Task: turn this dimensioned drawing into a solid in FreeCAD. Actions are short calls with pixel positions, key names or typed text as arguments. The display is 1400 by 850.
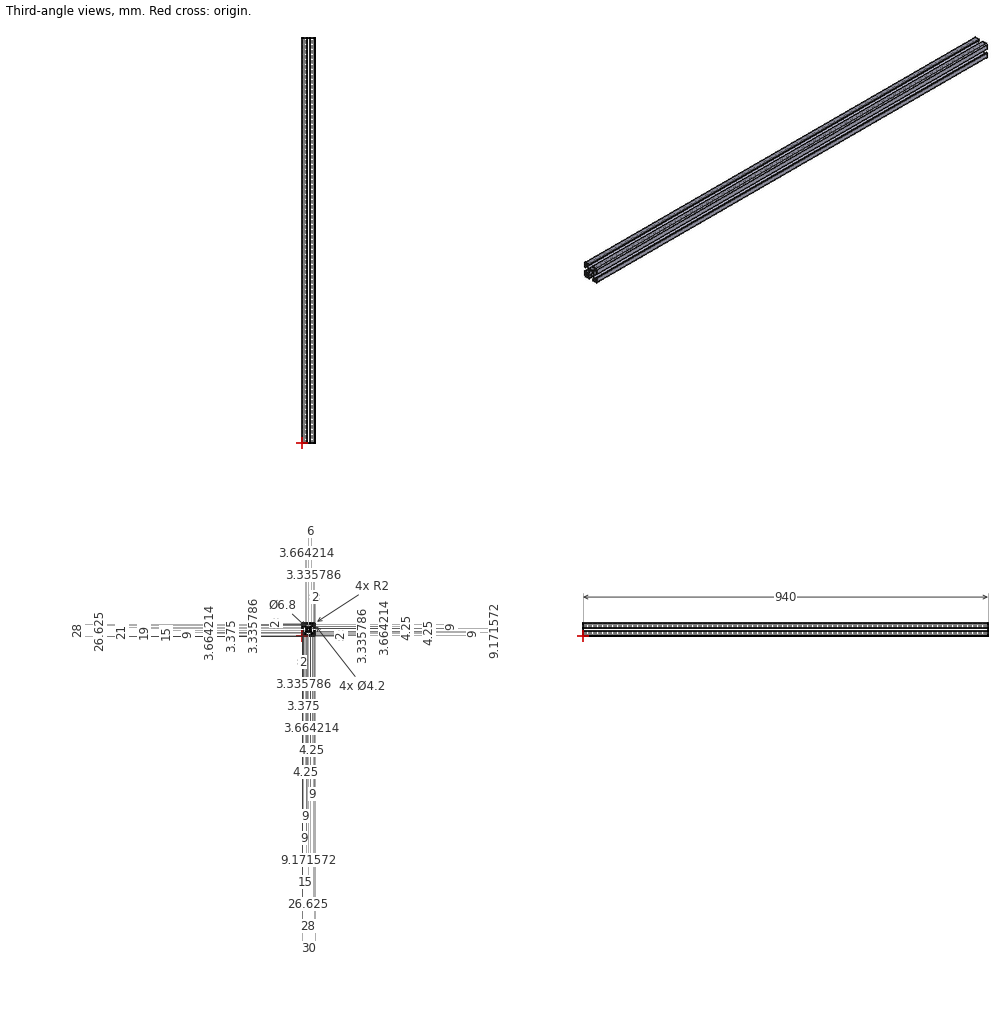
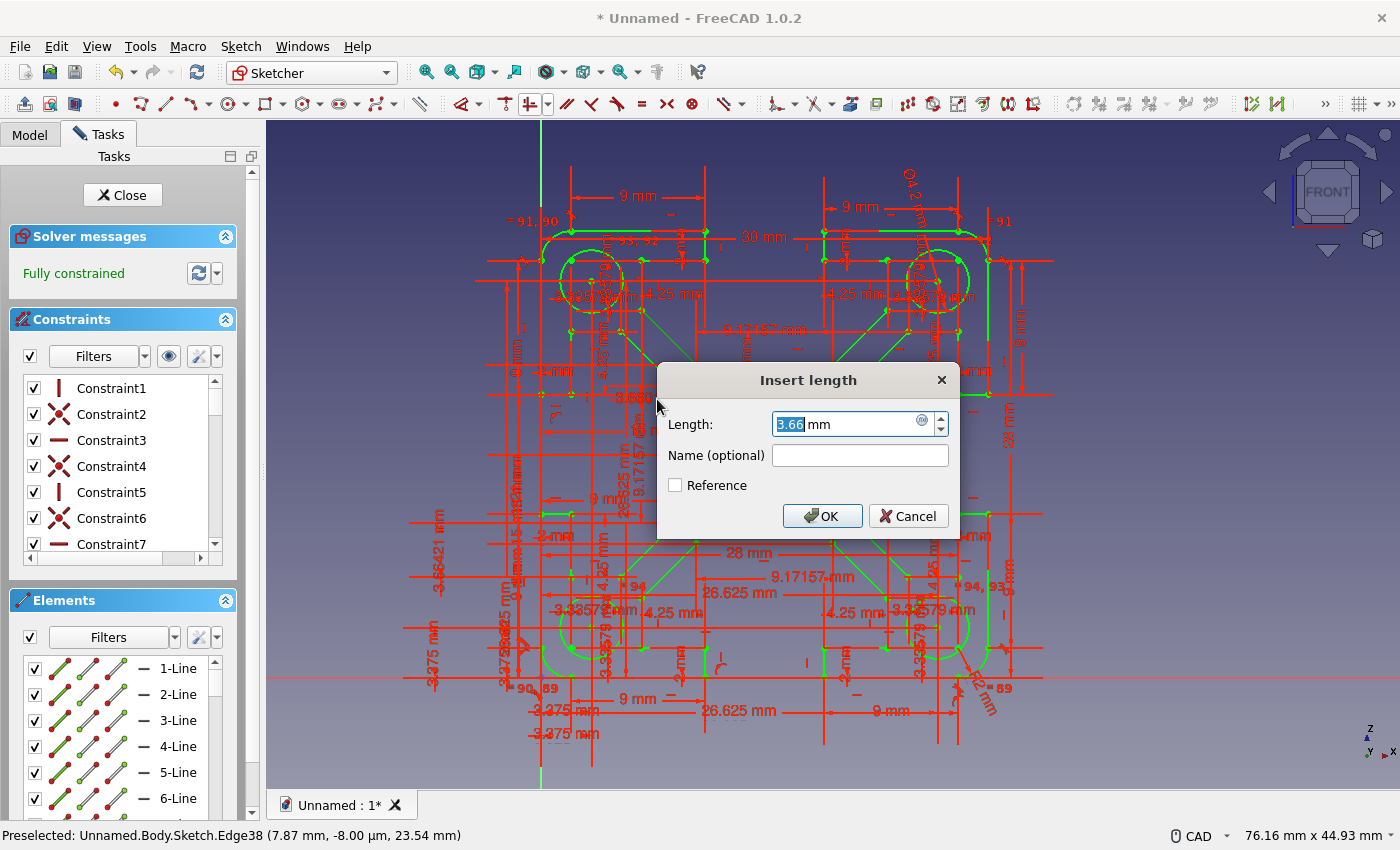
text(3.664214)
key(Return)
key(Escape)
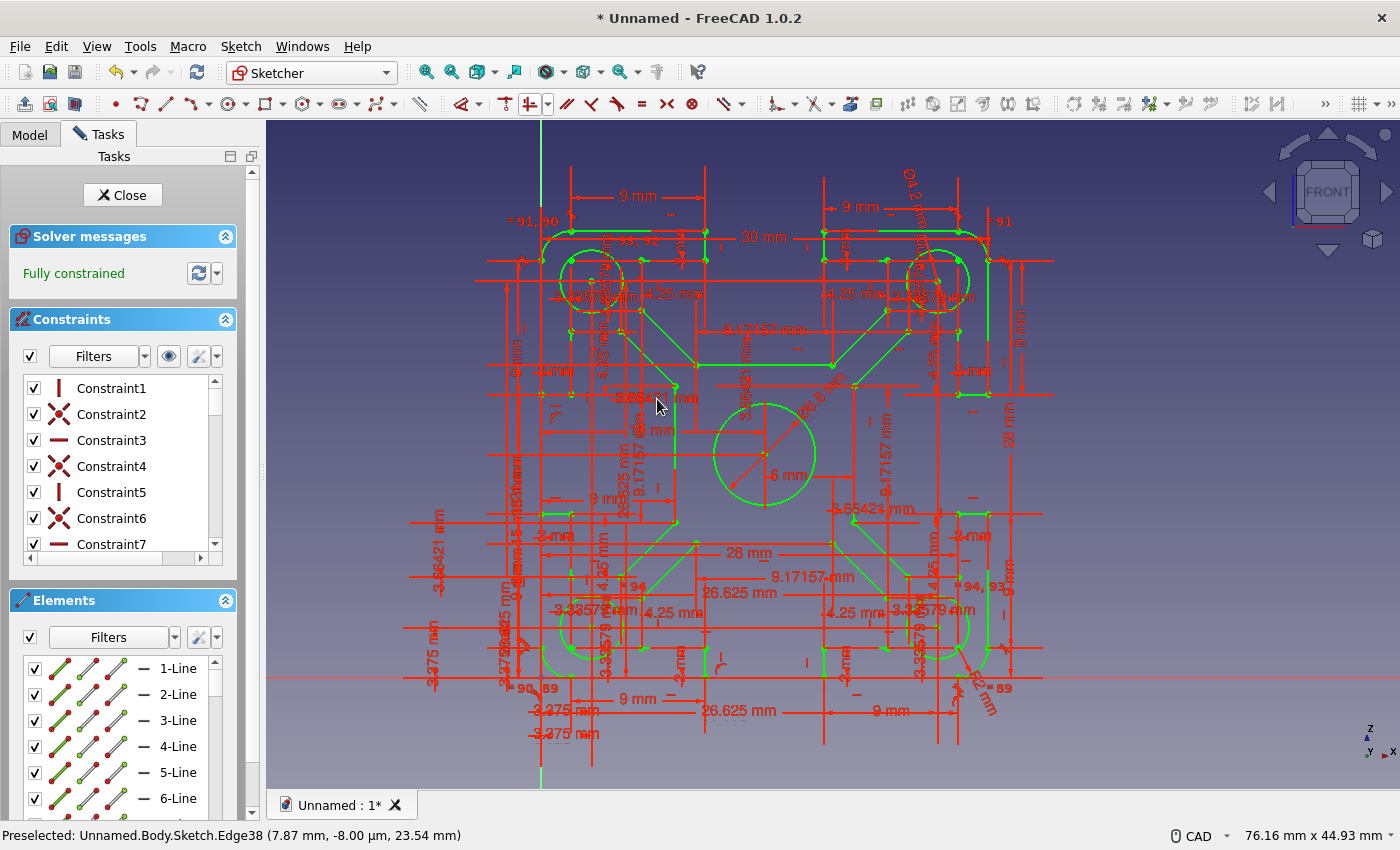
click(123, 195)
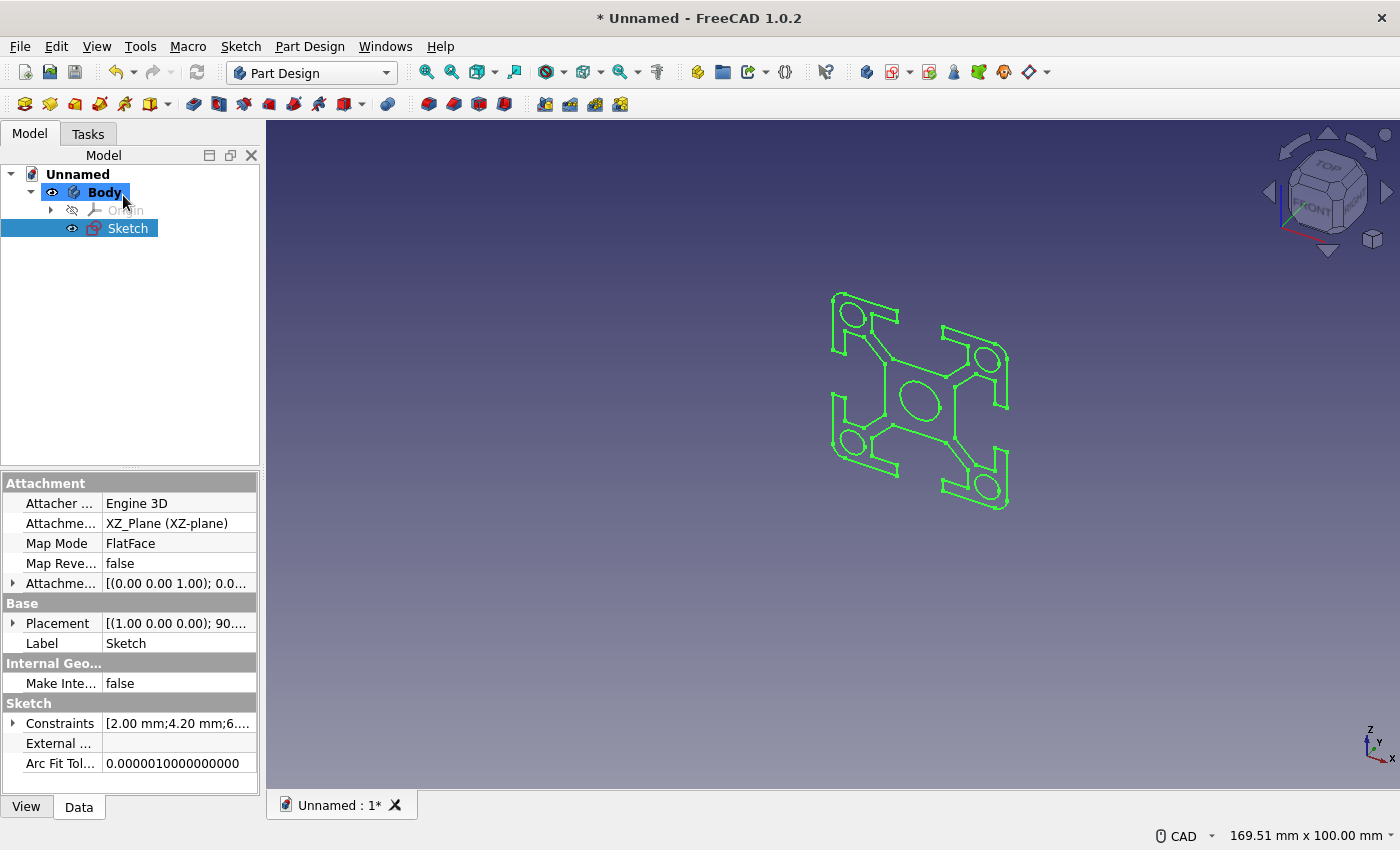
click(25, 104)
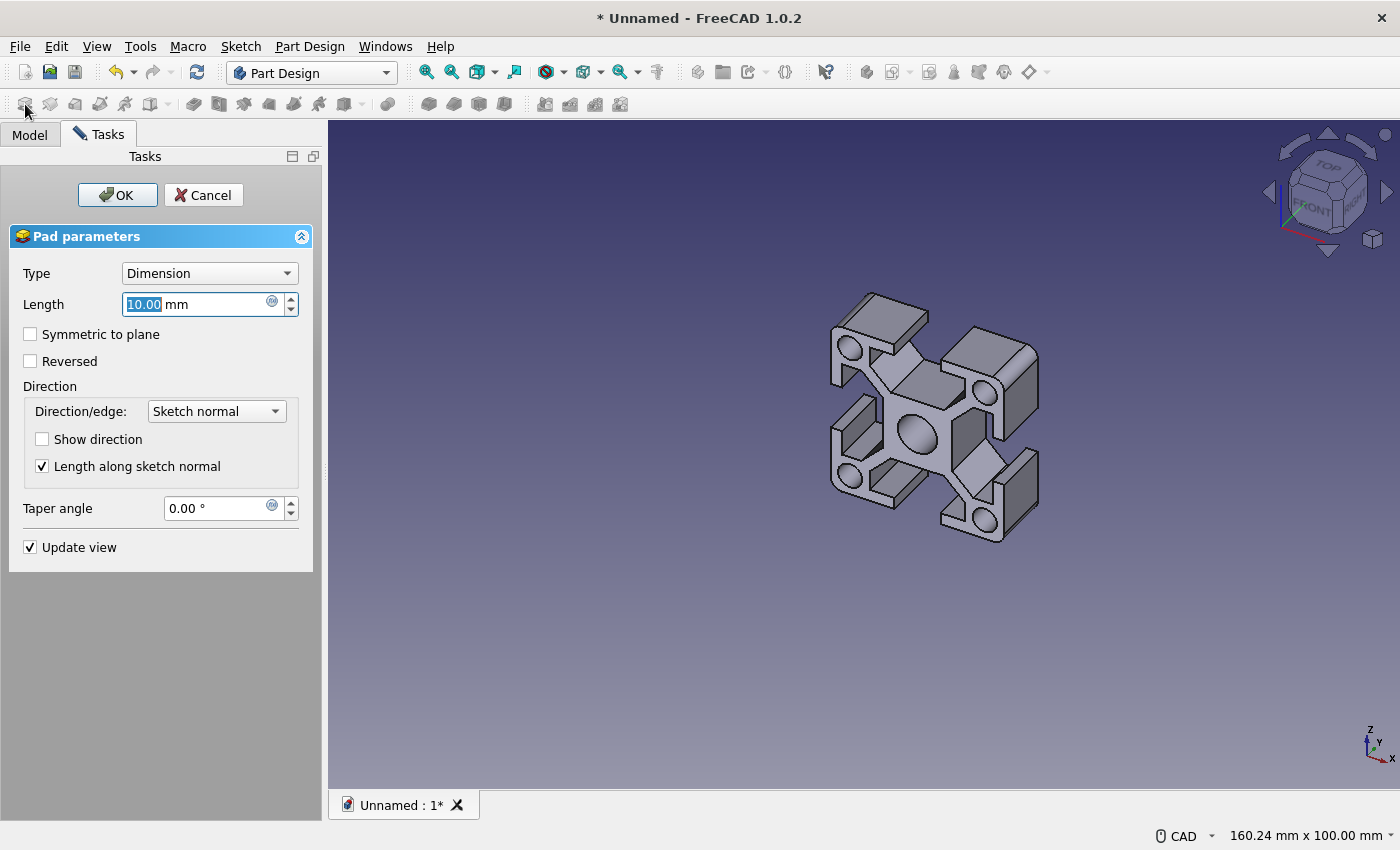
text(940)
key(Tab)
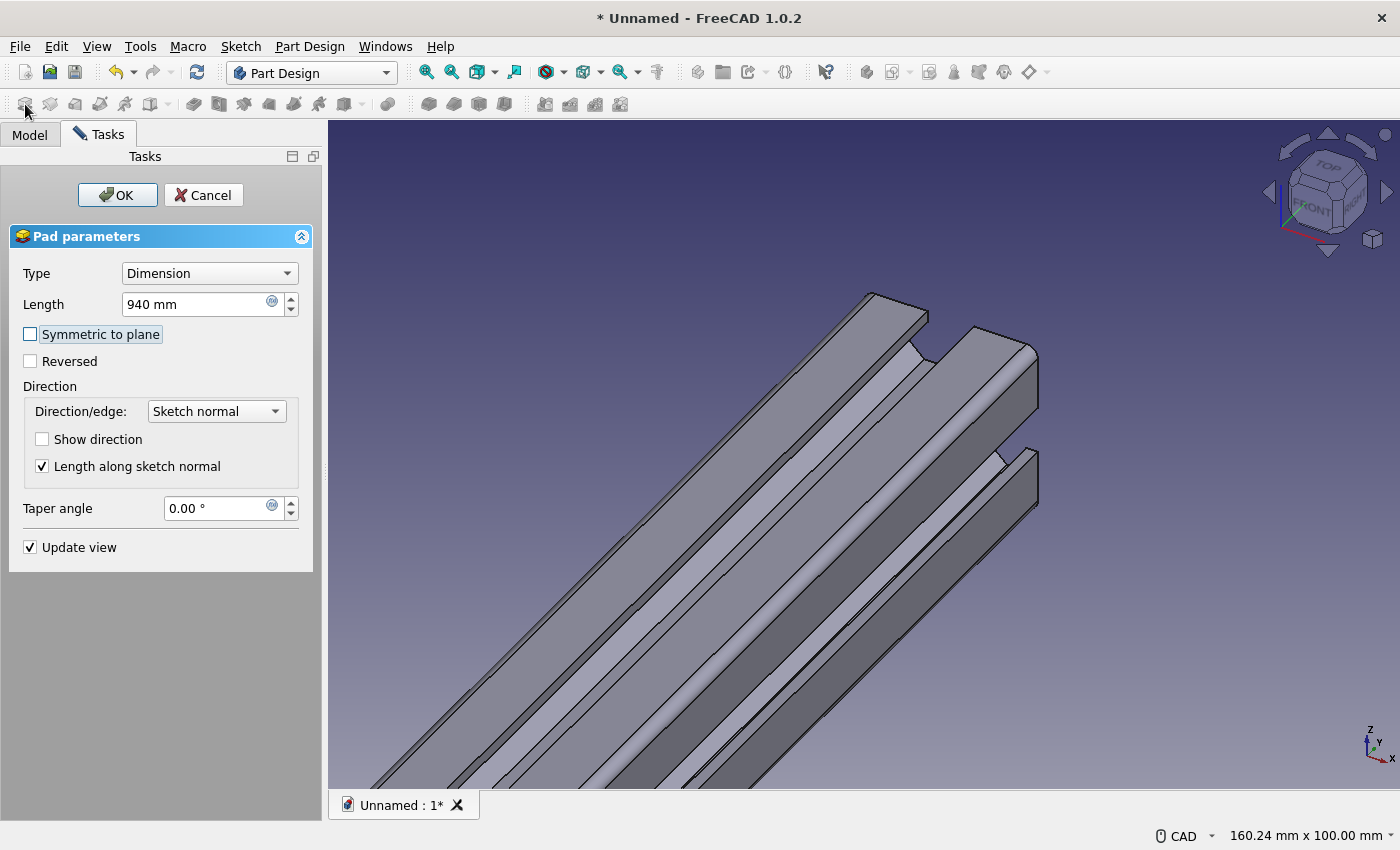
click(31, 361)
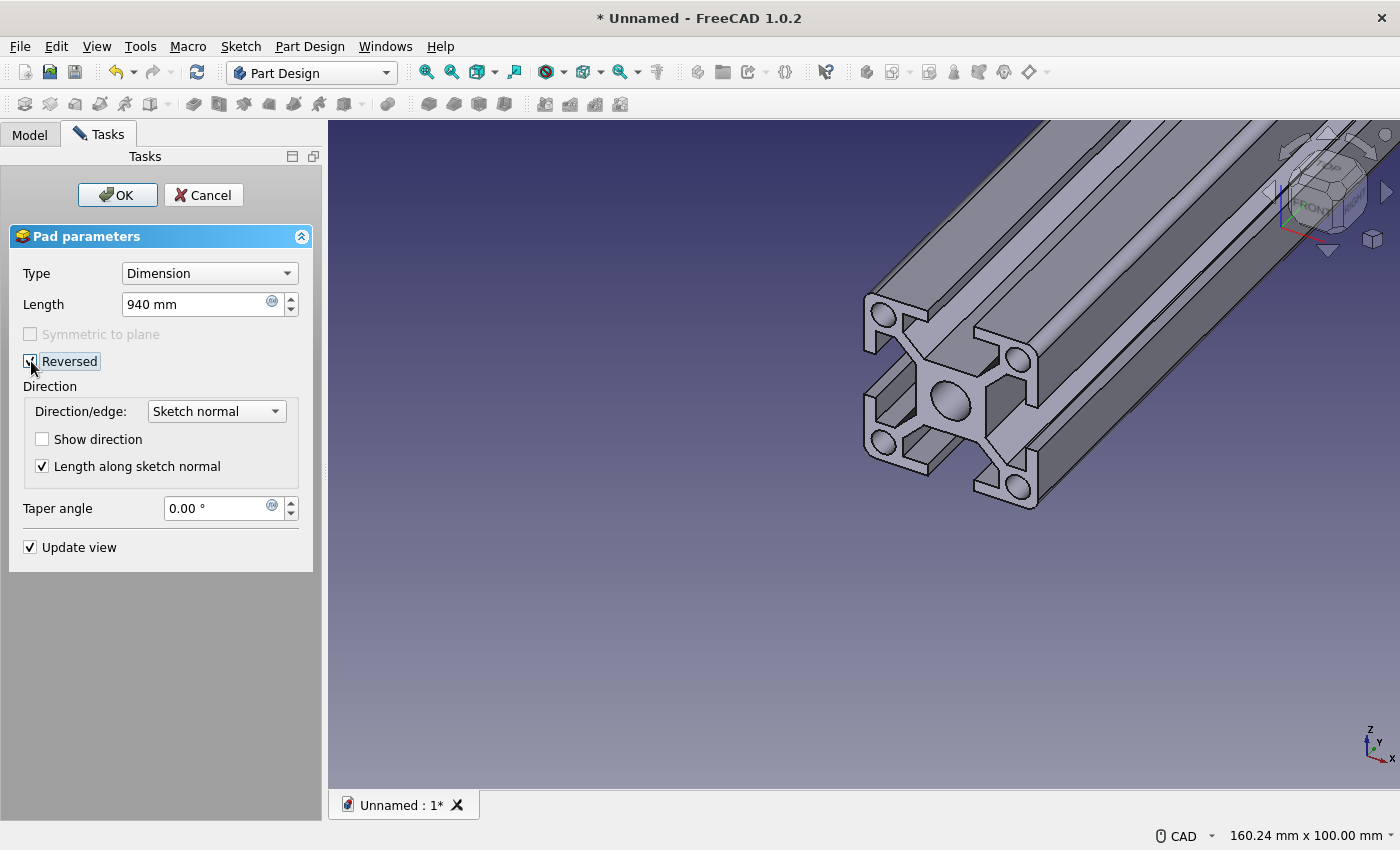
click(118, 195)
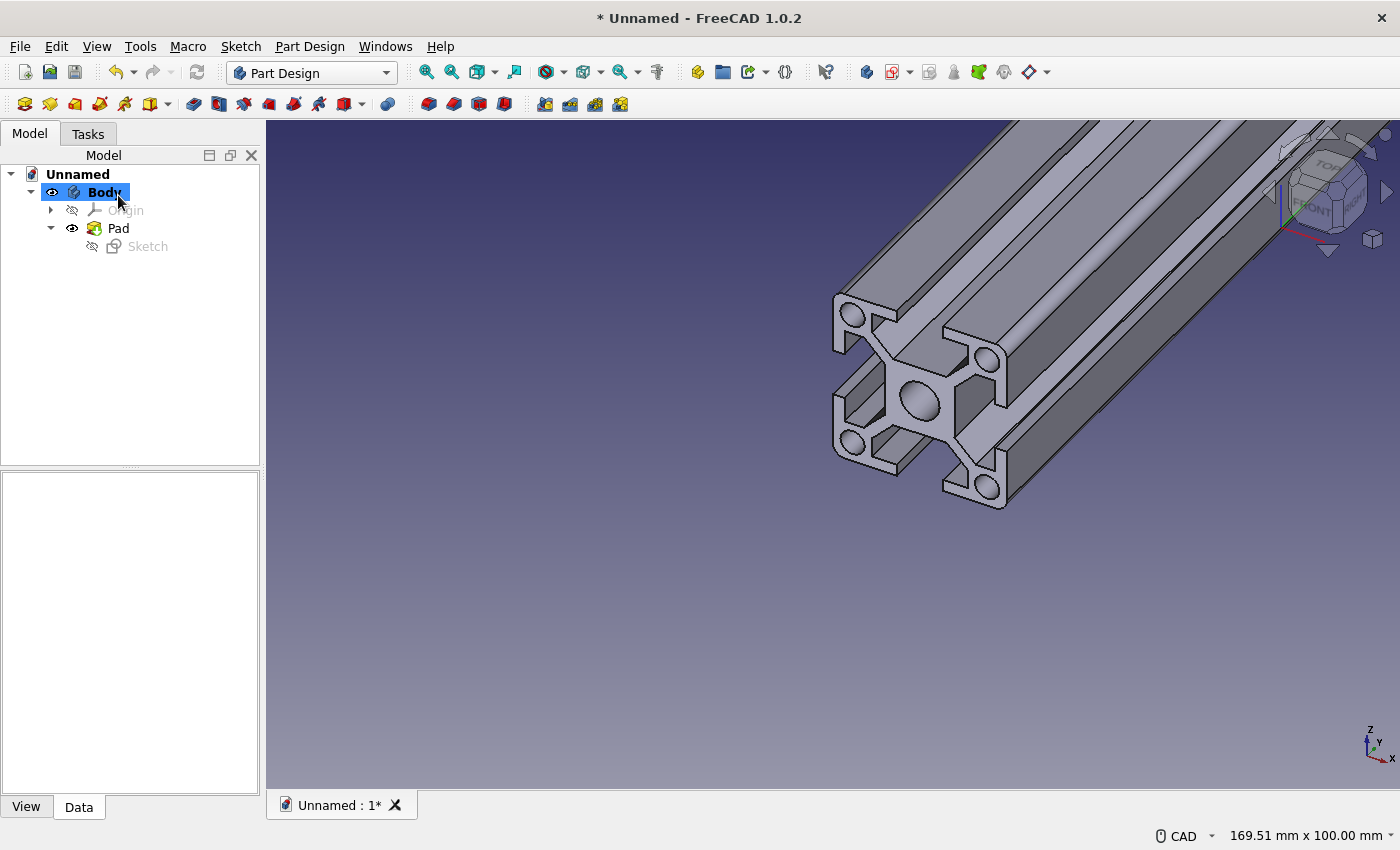
key(0)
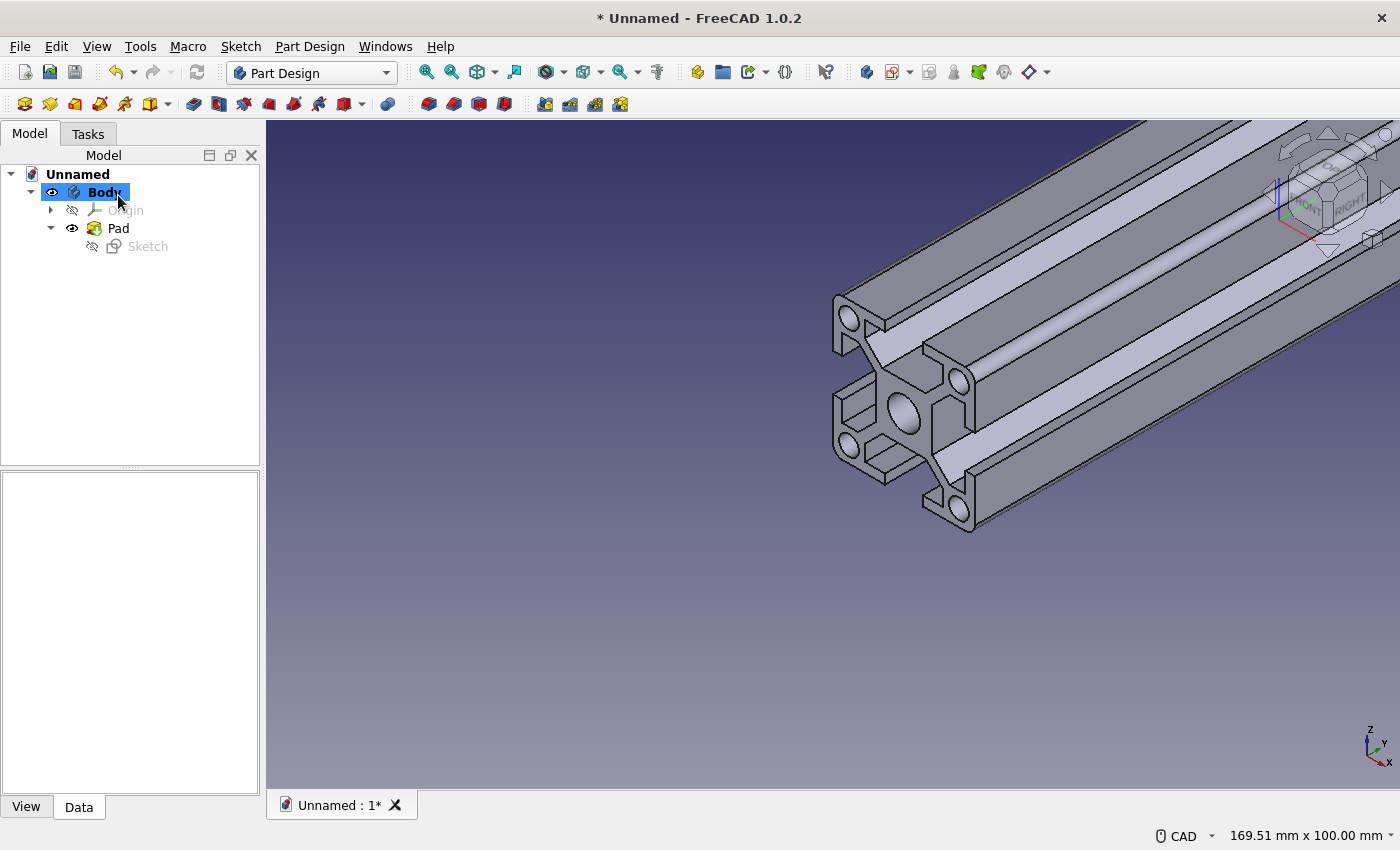
click(427, 72)